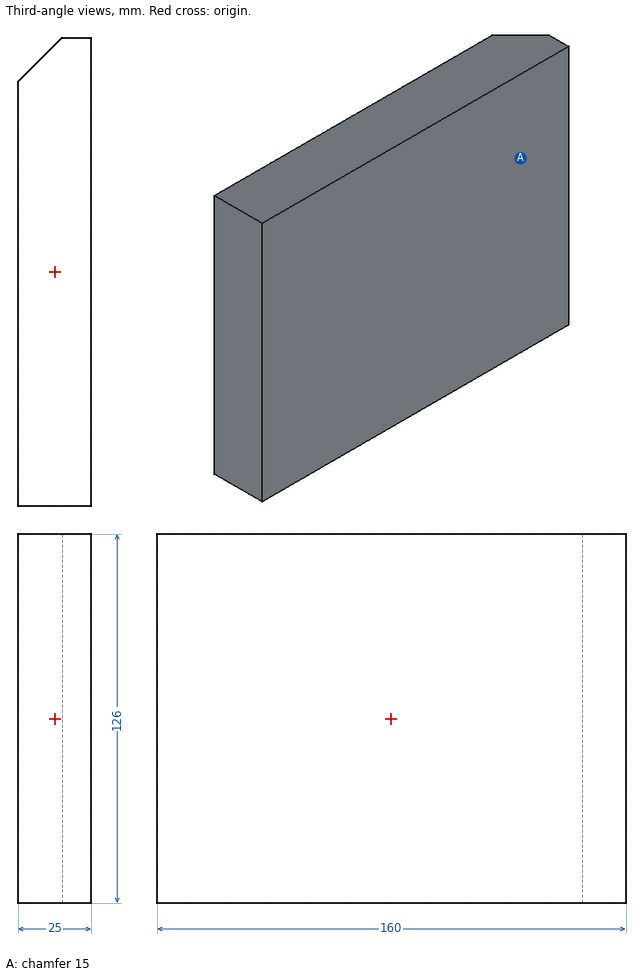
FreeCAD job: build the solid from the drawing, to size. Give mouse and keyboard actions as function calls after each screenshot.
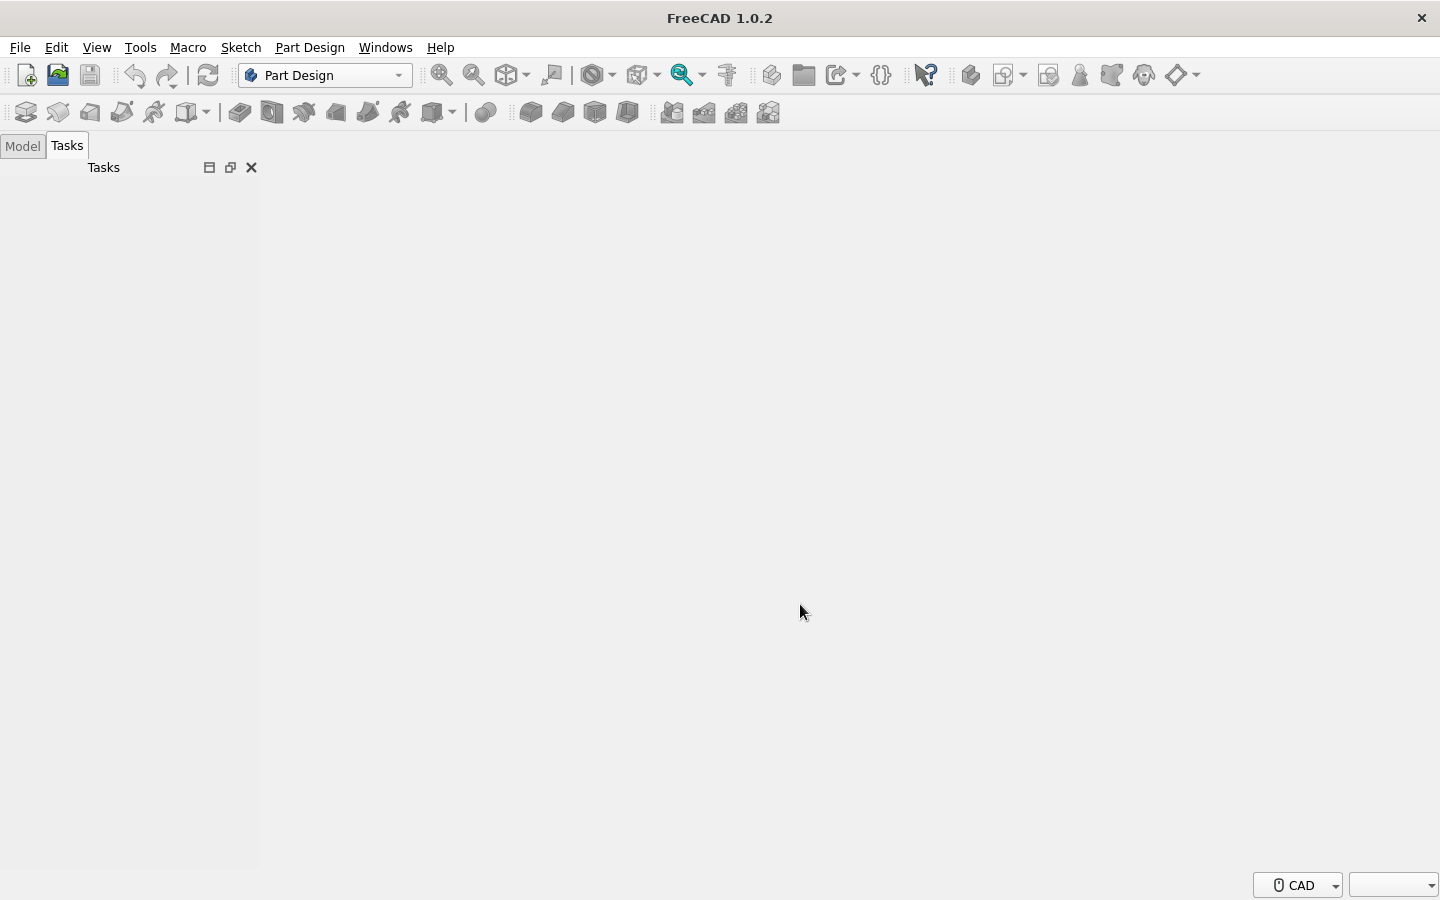
click(26, 76)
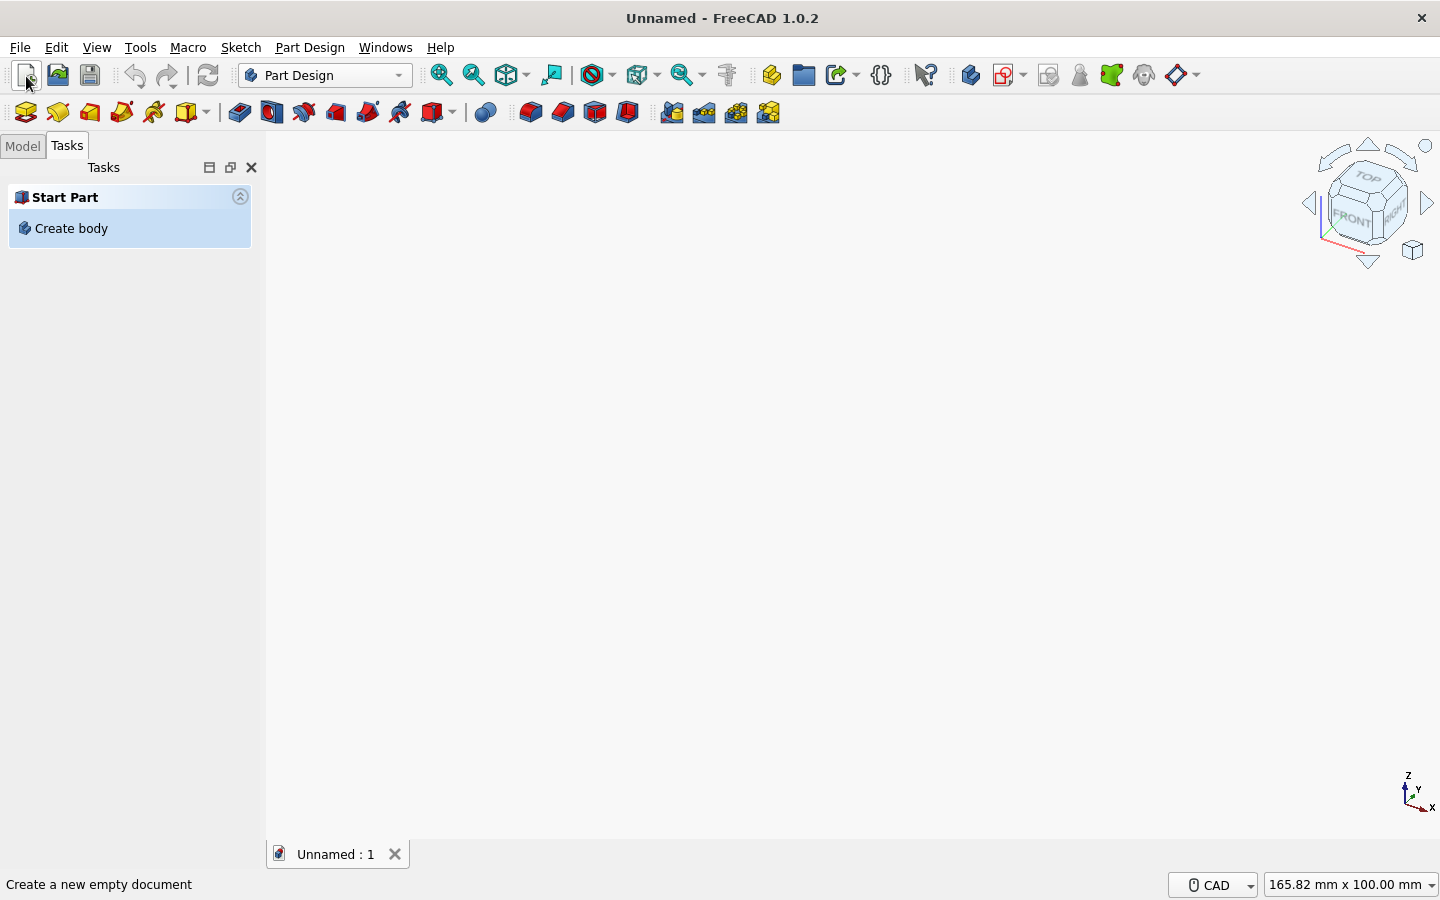
click(1004, 76)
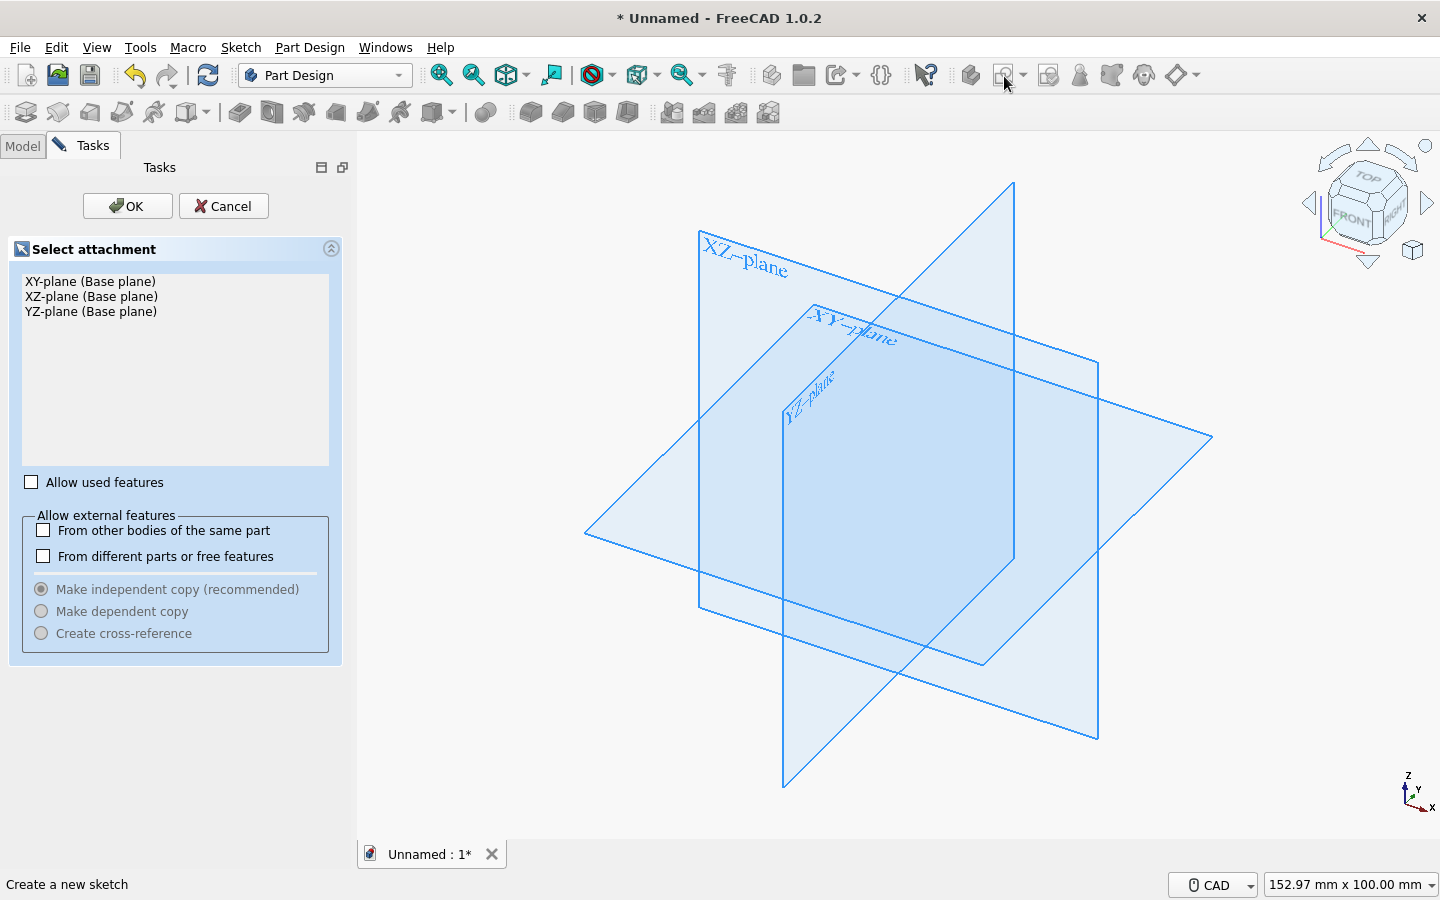
click(82, 296)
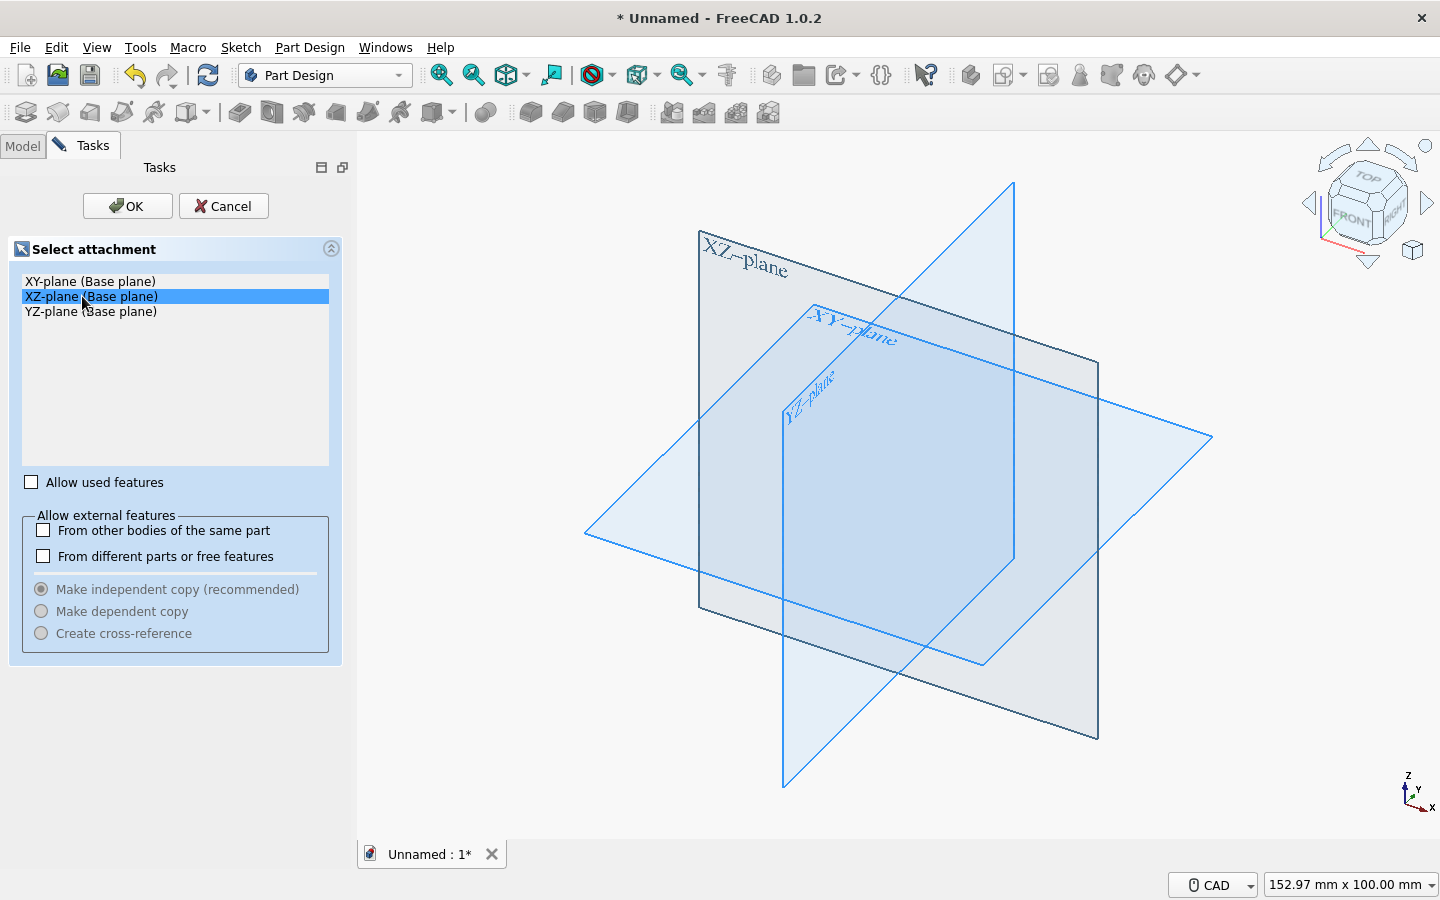
click(128, 206)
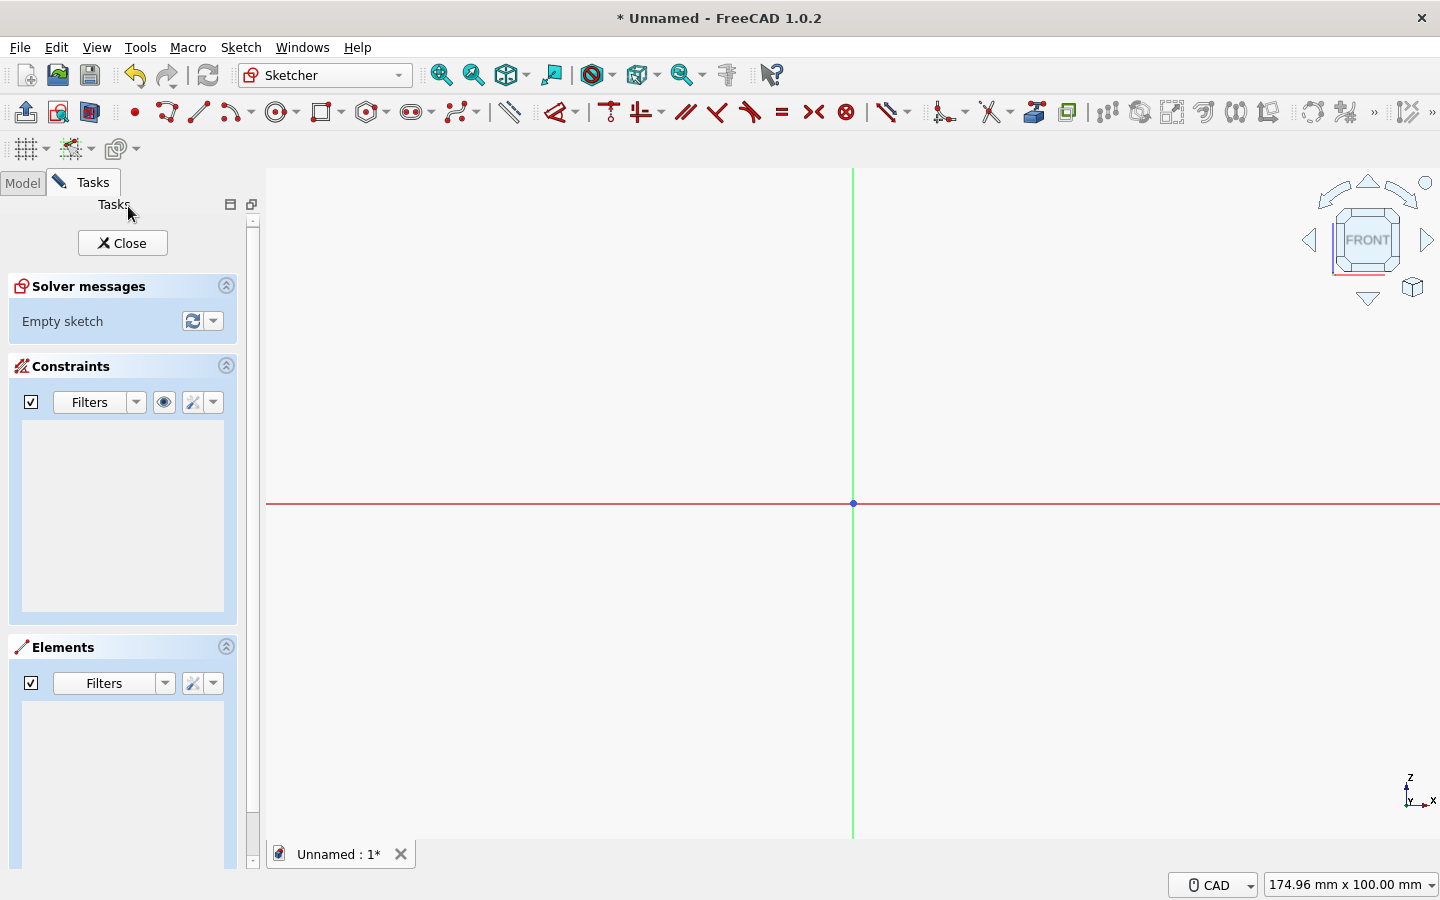
scroll(701, 504, down, 3)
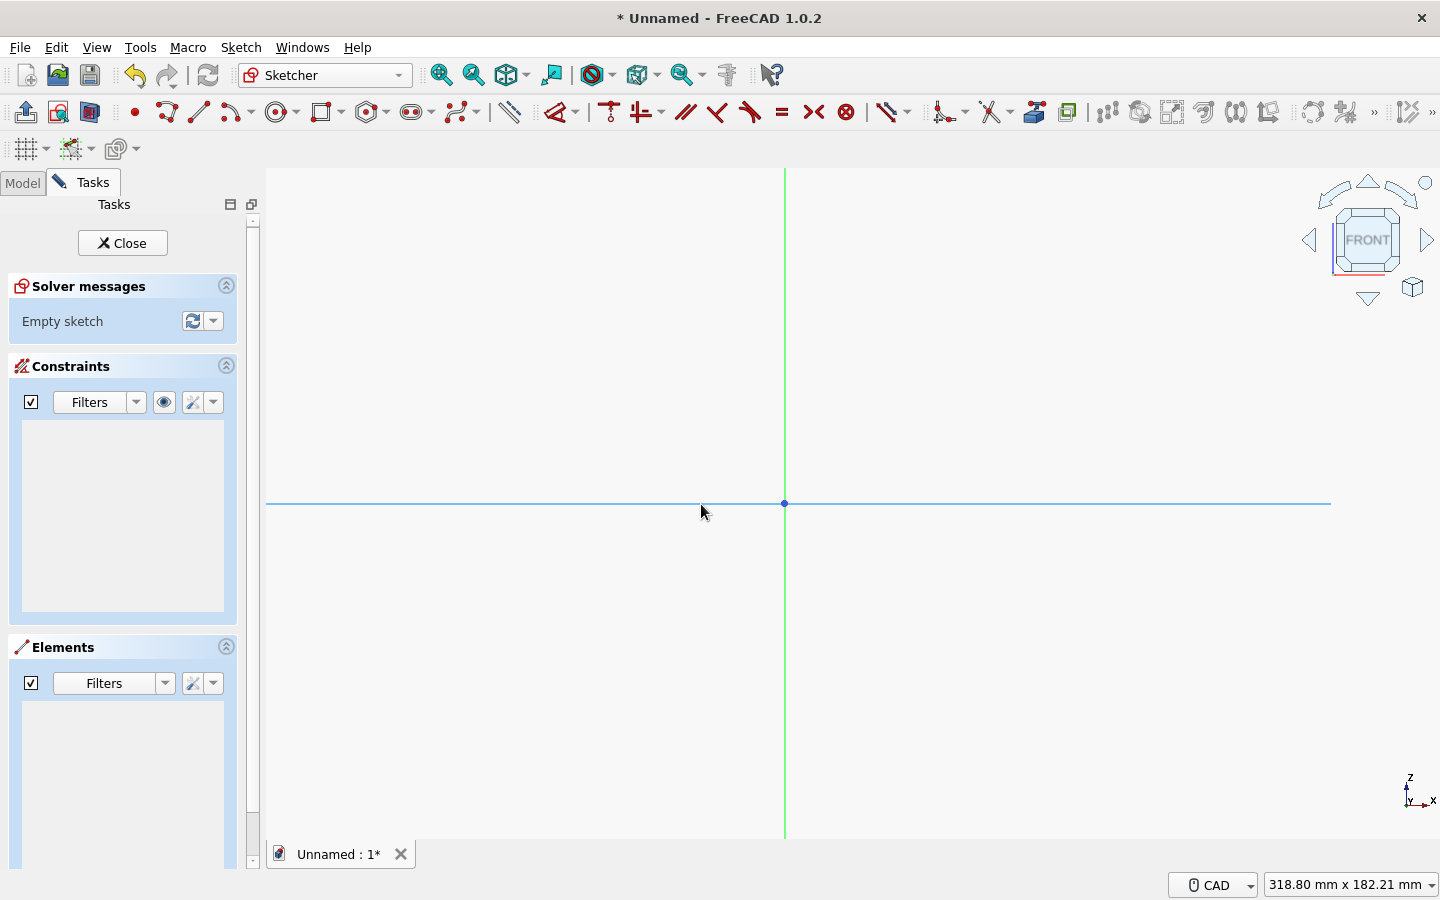
key(g)
key(v)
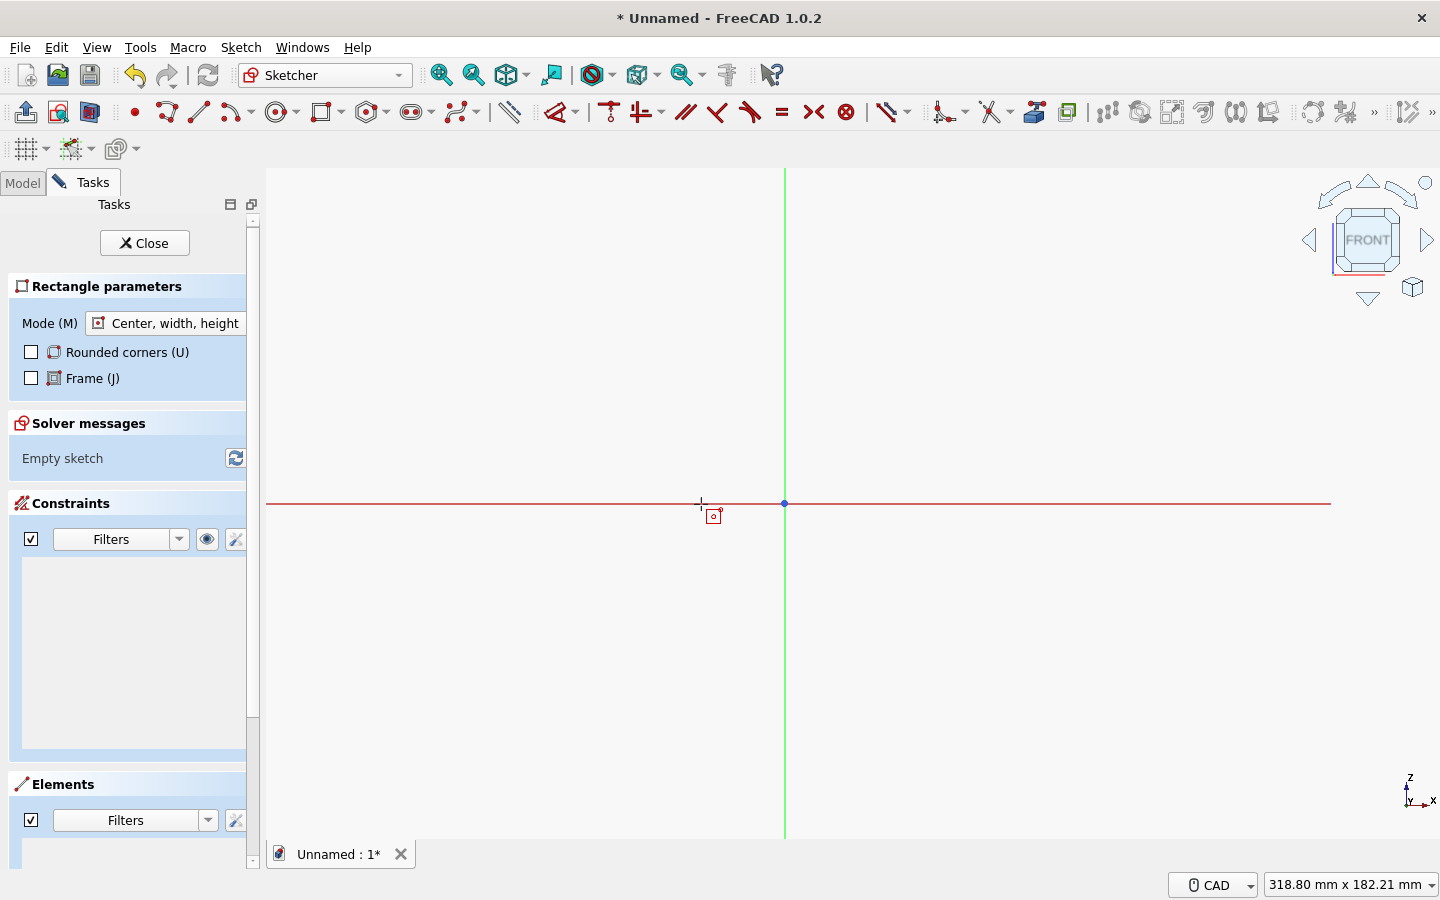
click(785, 504)
move(831, 272)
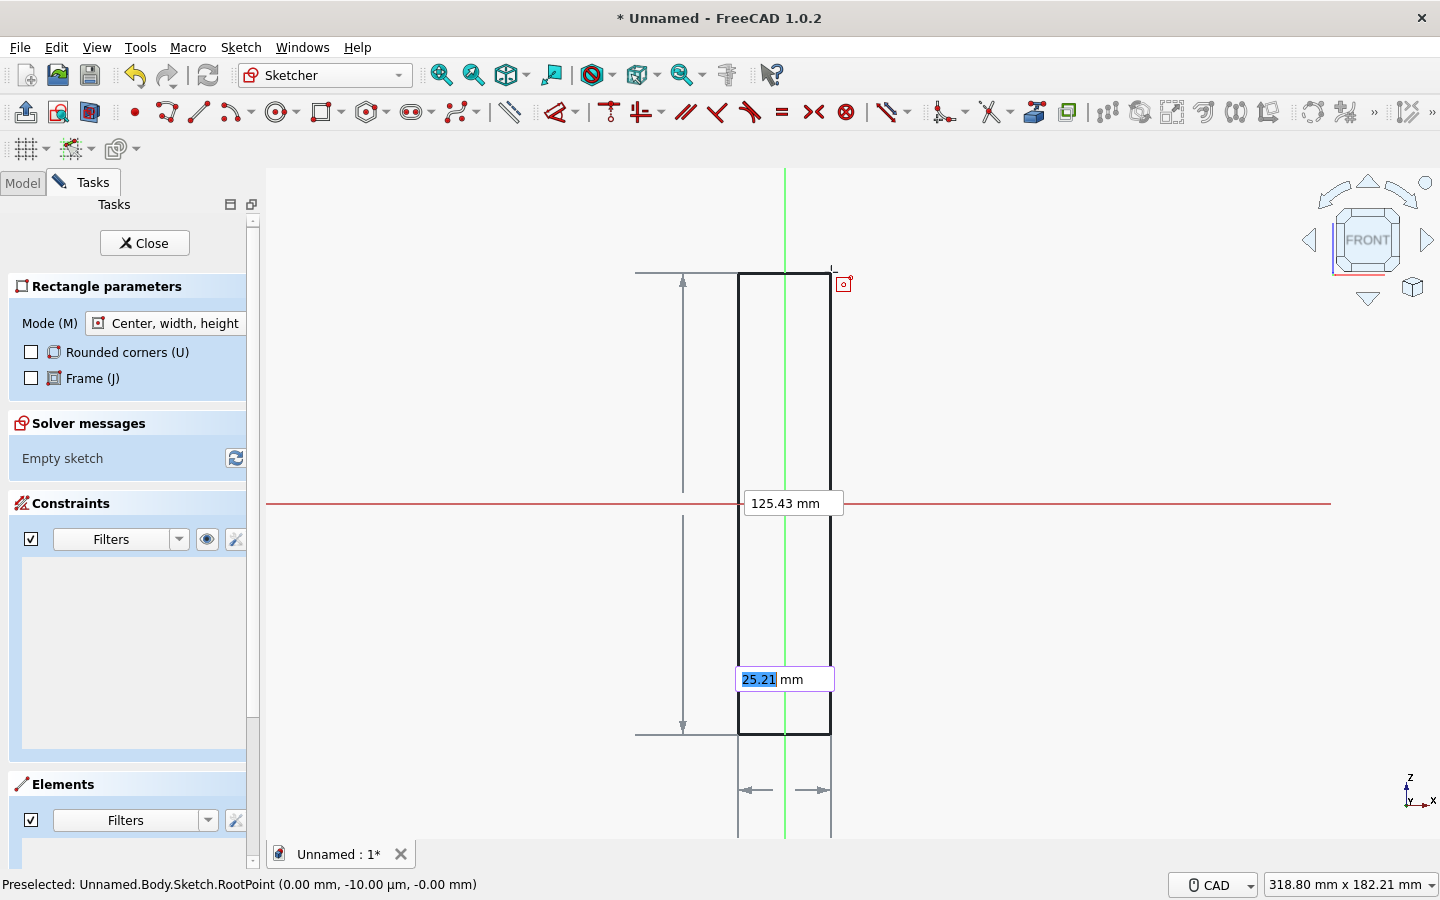
text(25)
key(Tab)
text(126)
key(Return)
key(Escape)